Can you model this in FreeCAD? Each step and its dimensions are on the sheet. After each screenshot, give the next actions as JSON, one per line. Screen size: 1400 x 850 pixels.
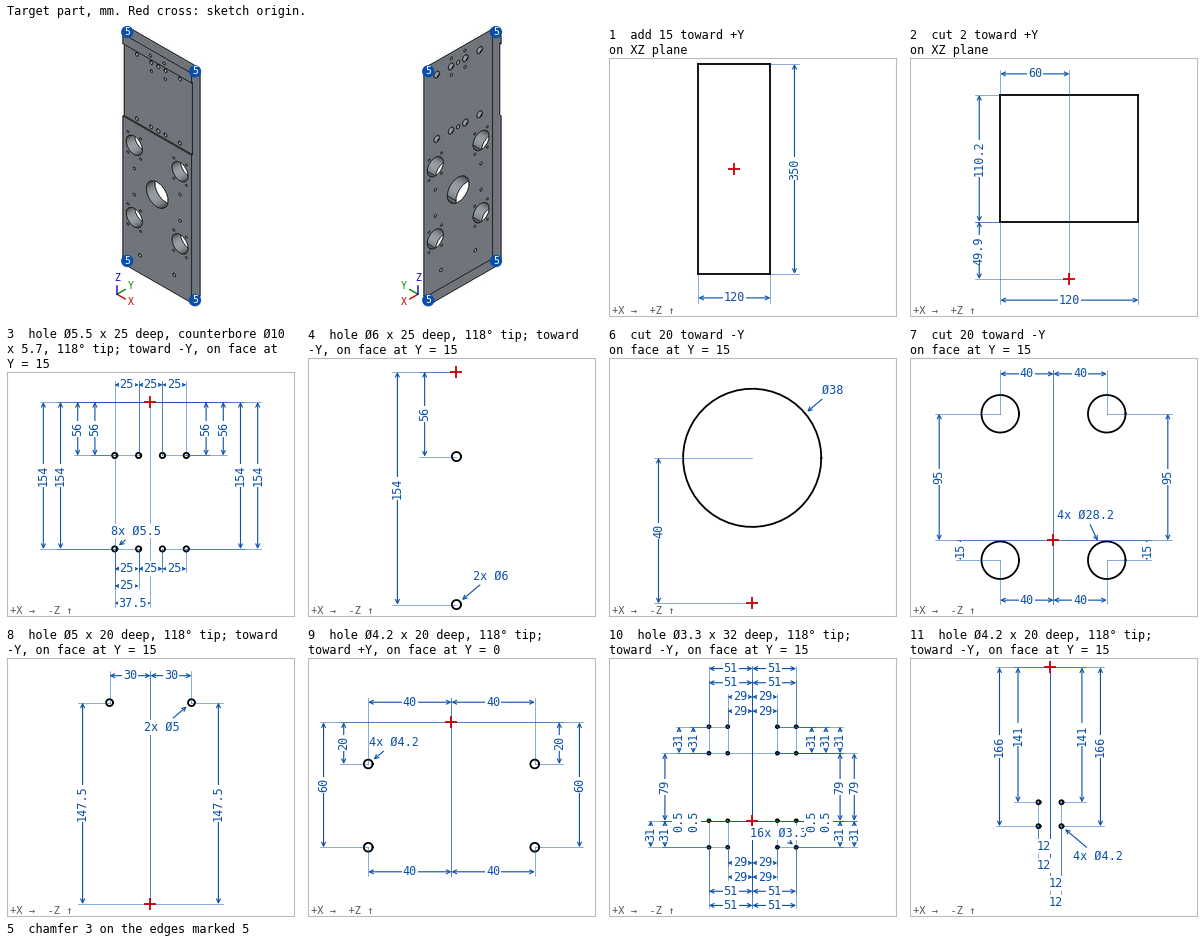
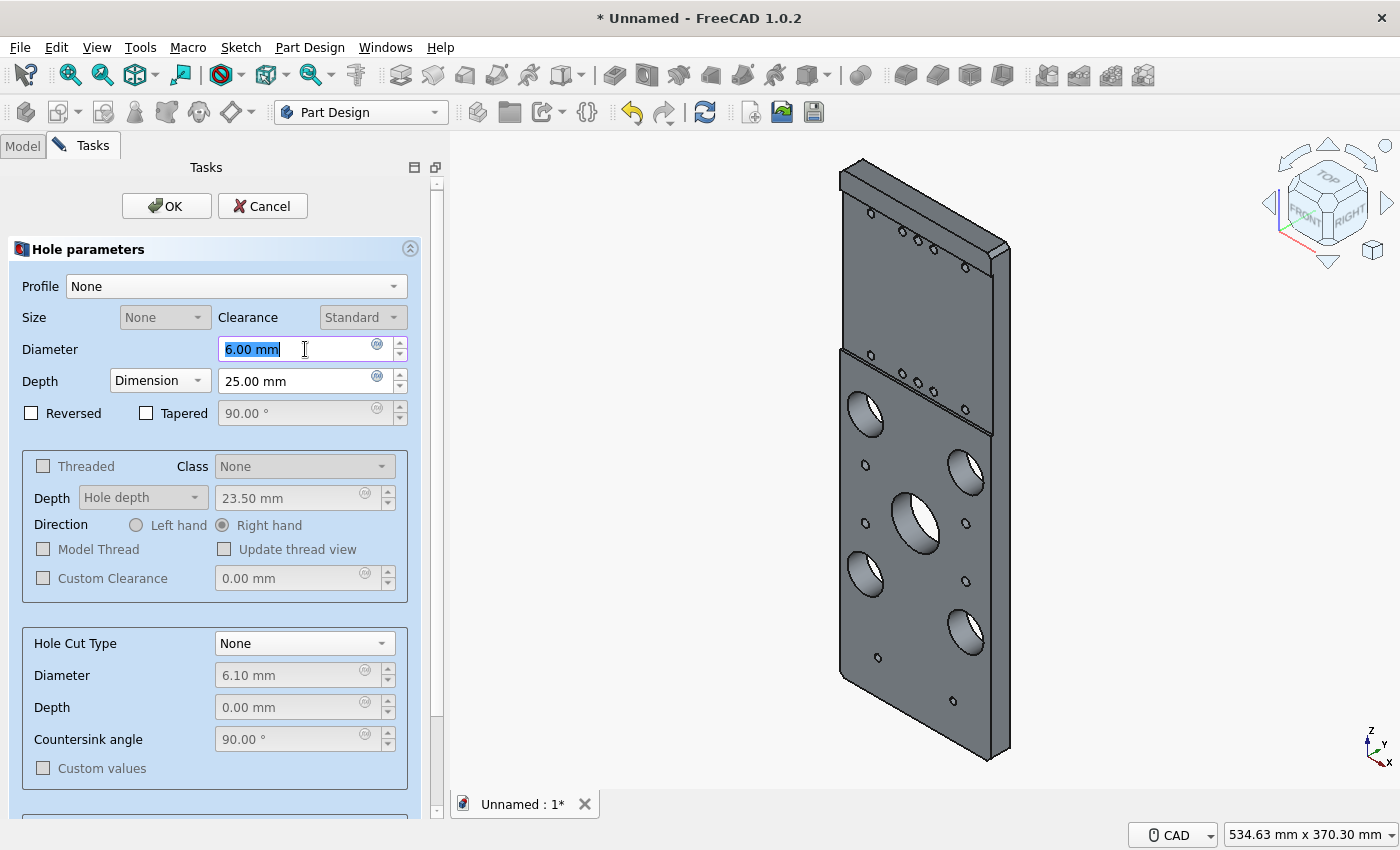
{"action": "type", "text": "4.2"}
{"action": "key", "text": "Tab"}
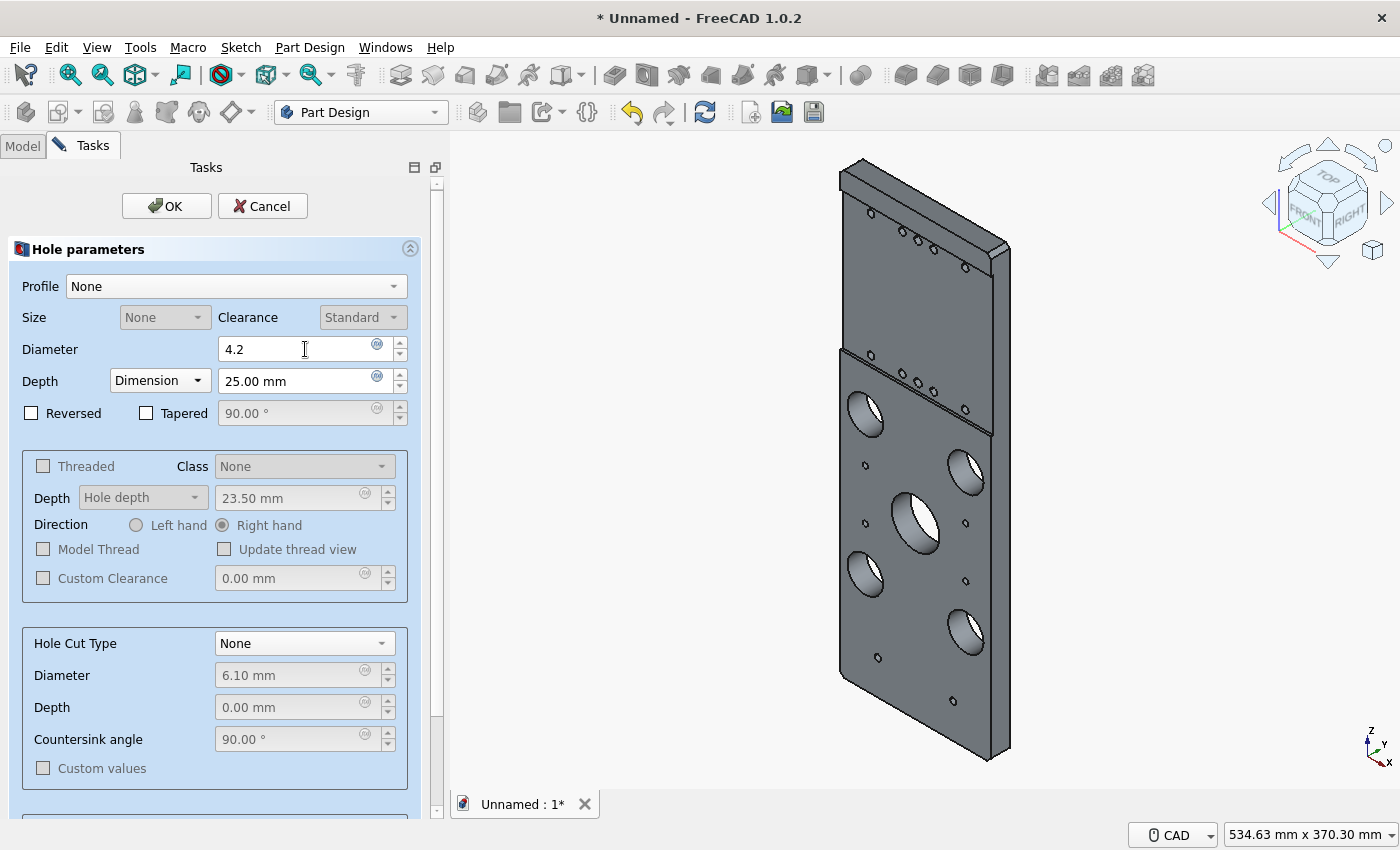
{"action": "triple_click", "coordinate": [305, 381]}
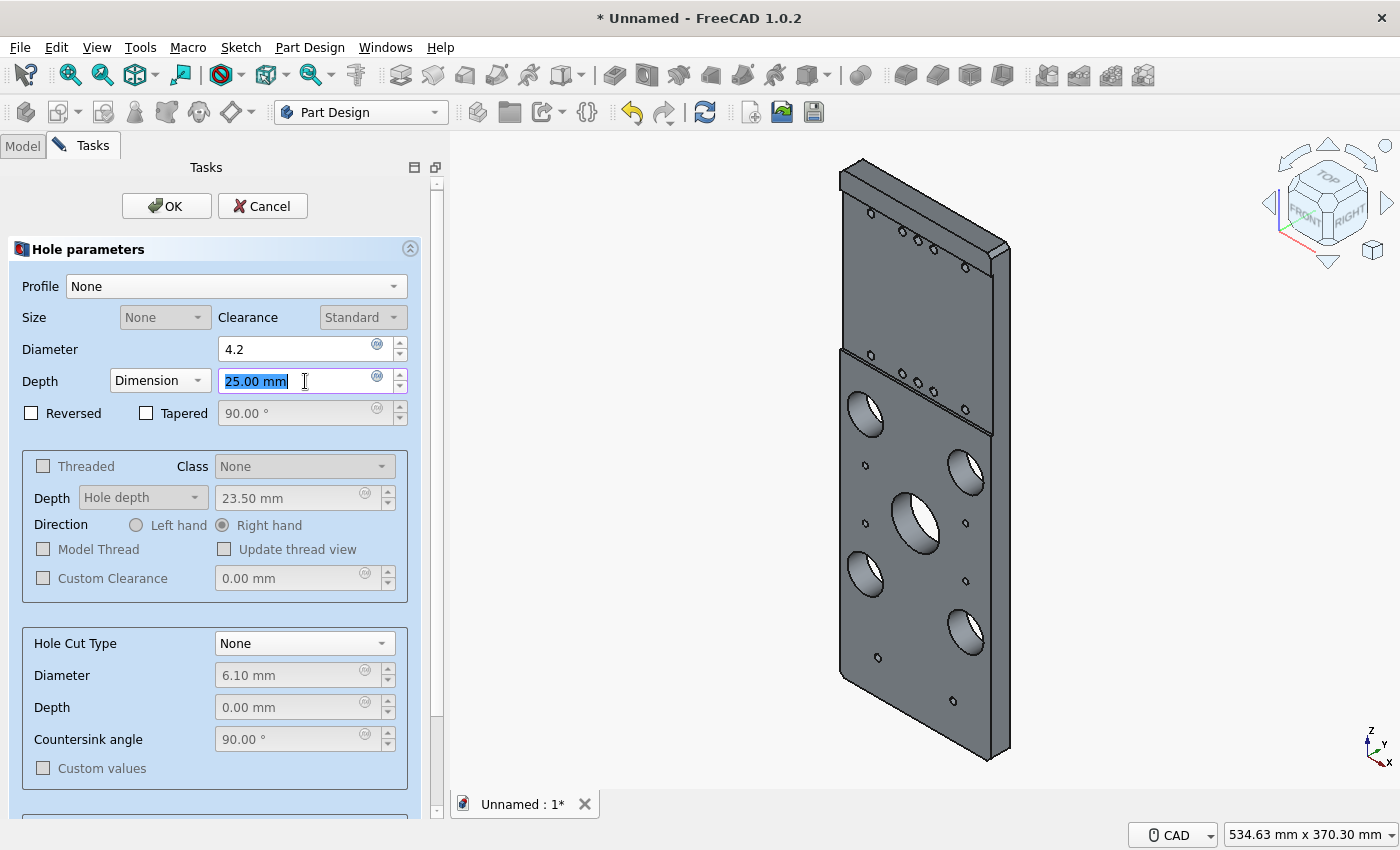
{"action": "type", "text": "20"}
{"action": "key", "text": "Tab"}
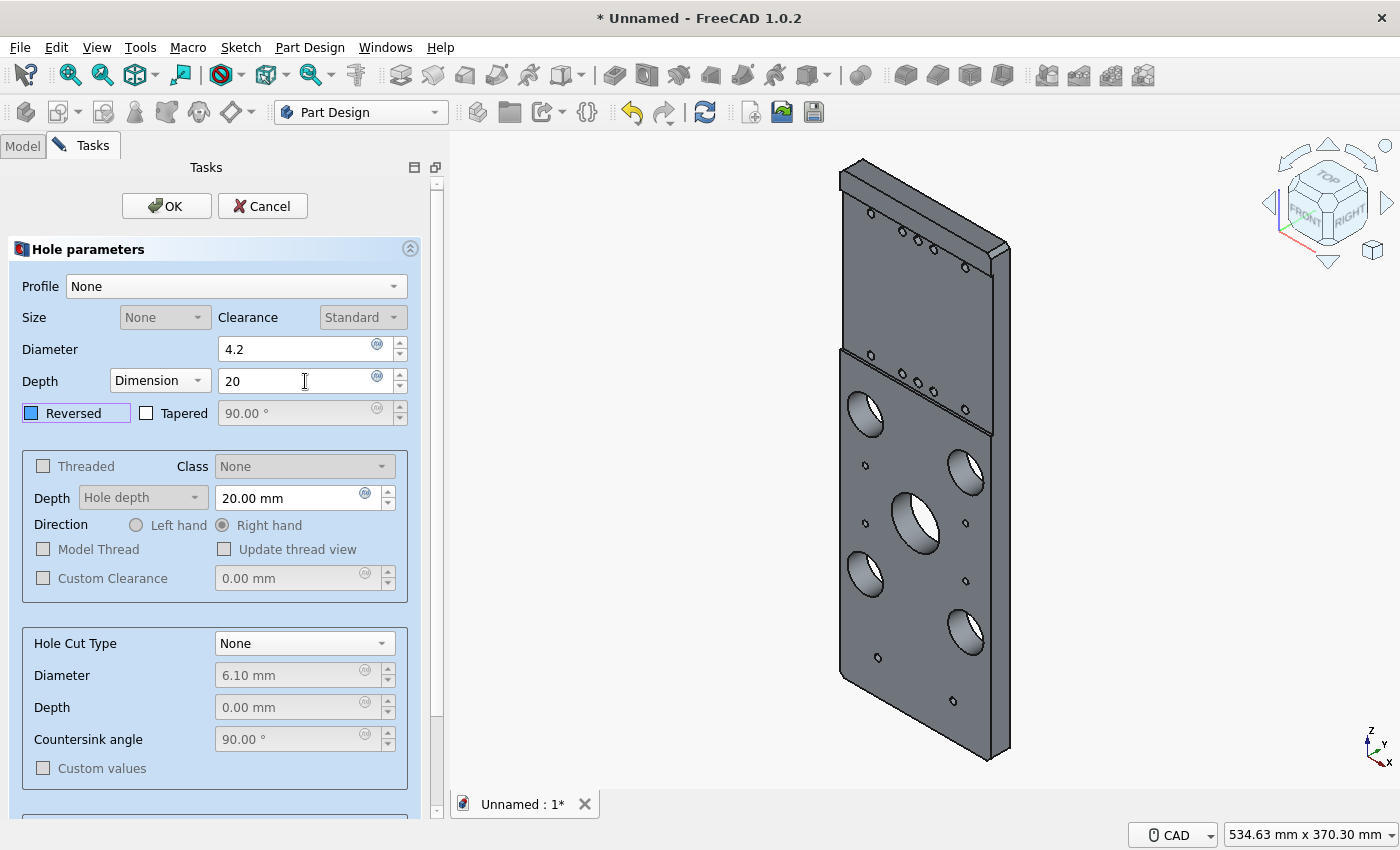
{"action": "left_click", "coordinate": [167, 206]}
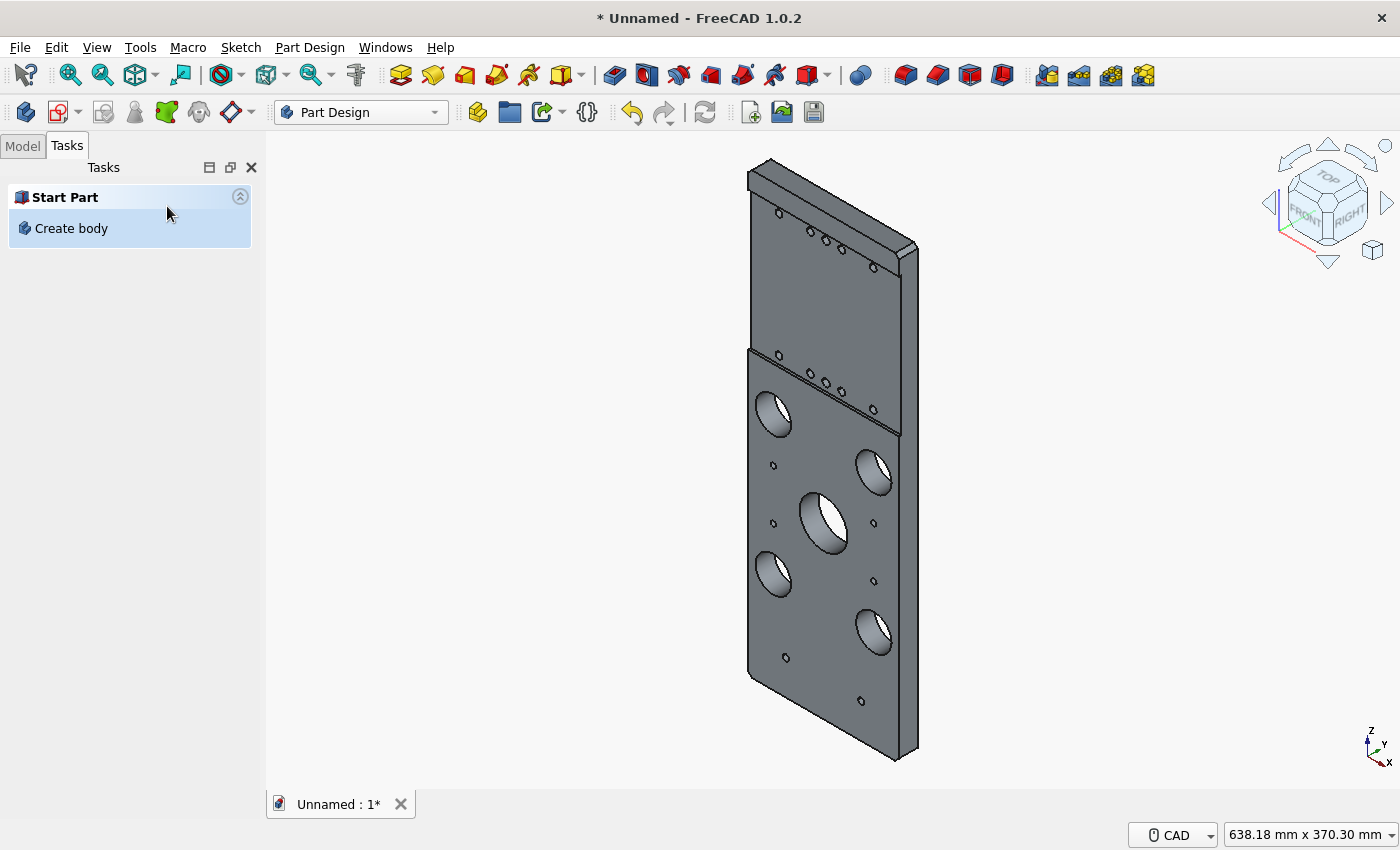
{"action": "key", "text": "4"}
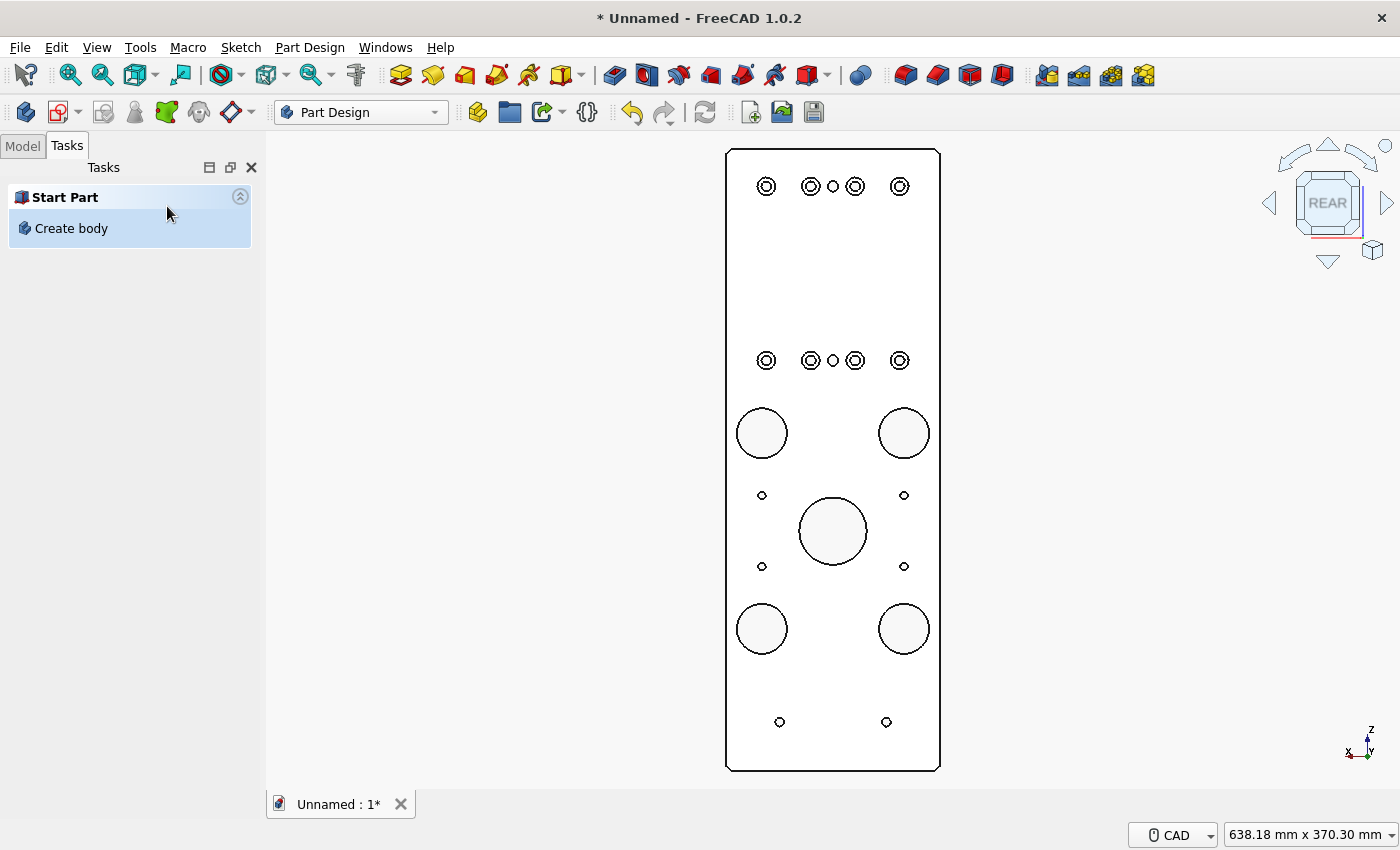
{"action": "left_click", "coordinate": [833, 281]}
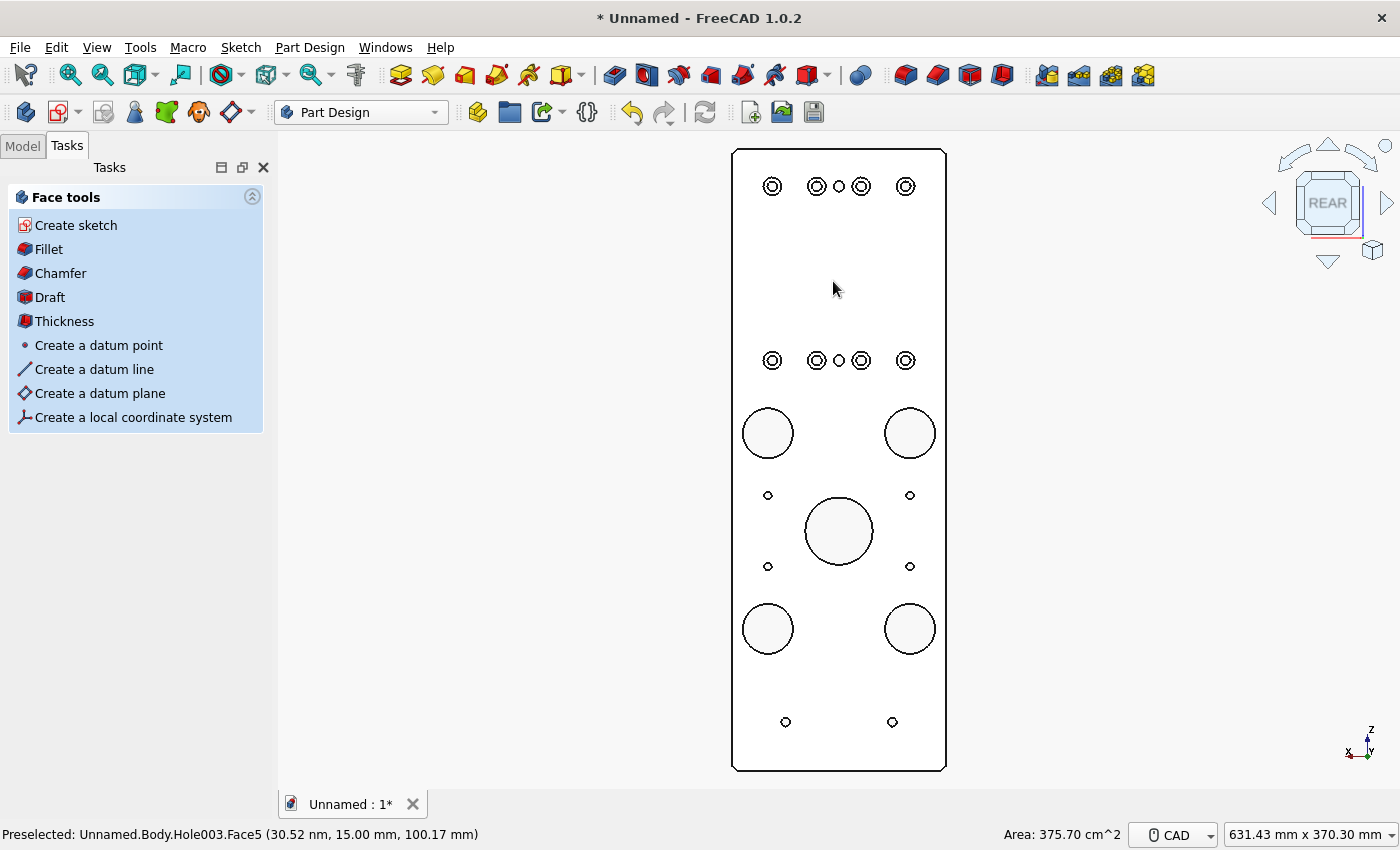
{"action": "left_click", "coordinate": [58, 112]}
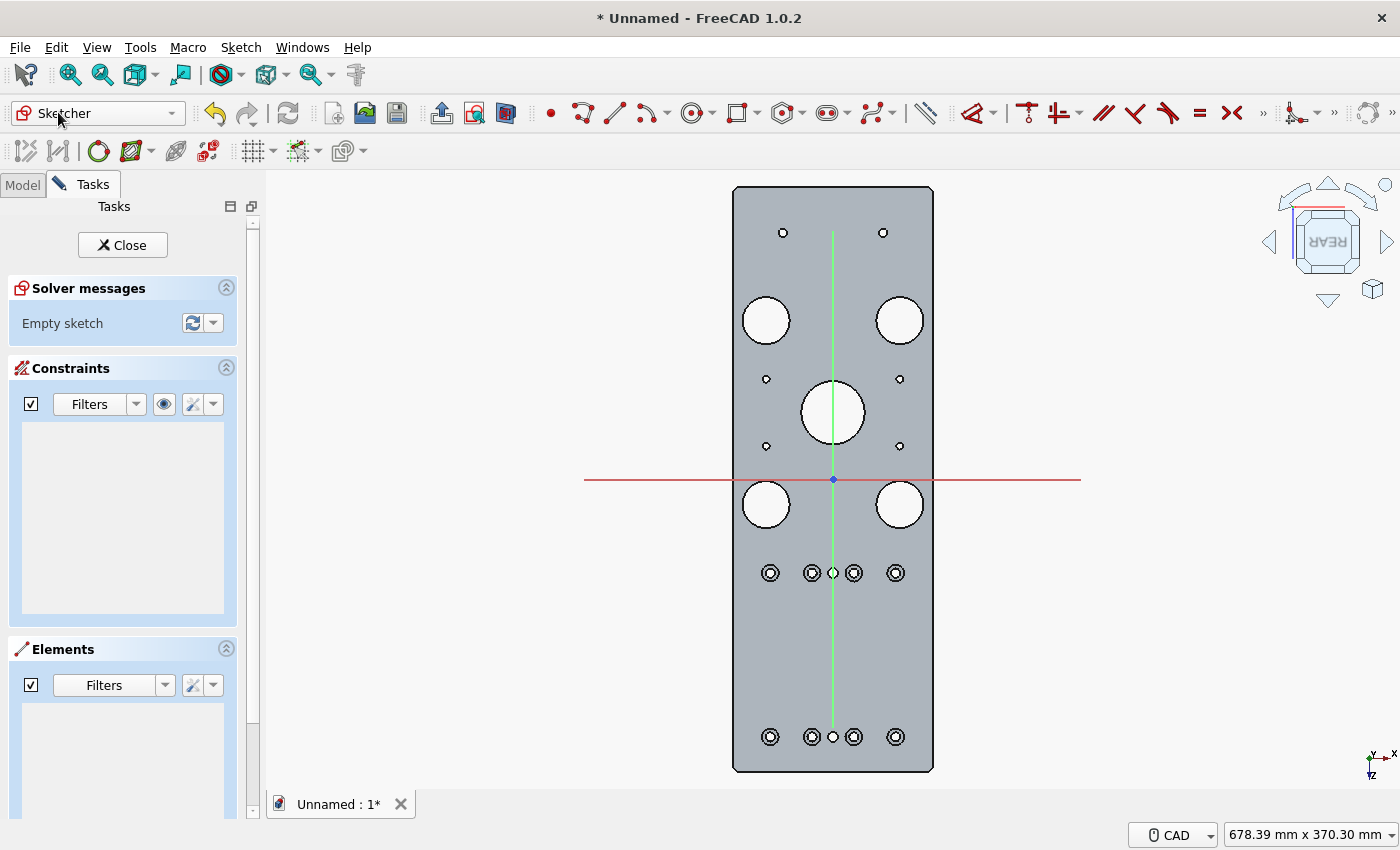
{"action": "scroll", "coordinate": [972, 277], "scroll_direction": "up", "scroll_amount": 2}